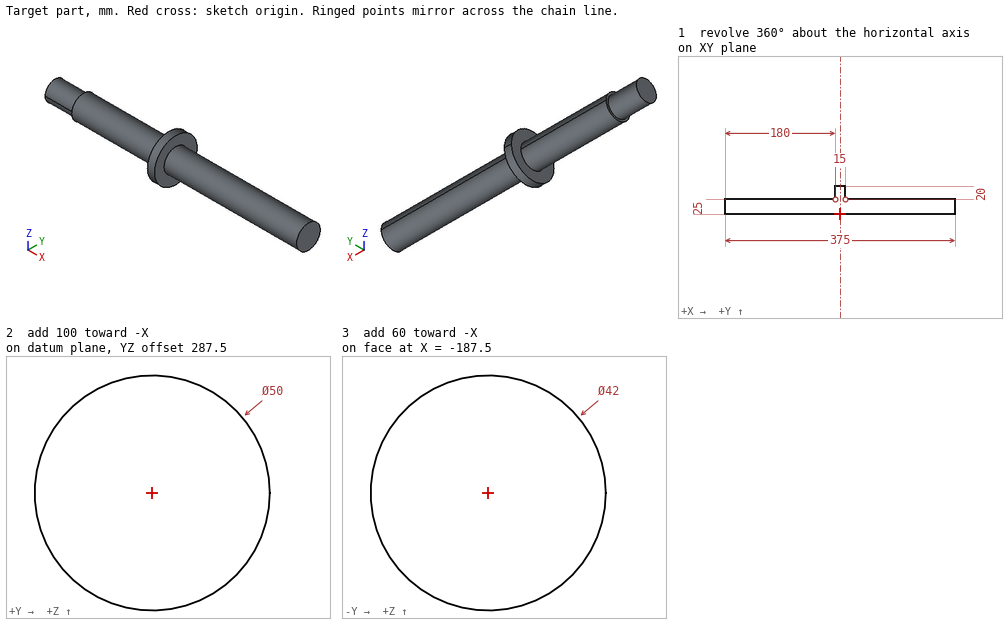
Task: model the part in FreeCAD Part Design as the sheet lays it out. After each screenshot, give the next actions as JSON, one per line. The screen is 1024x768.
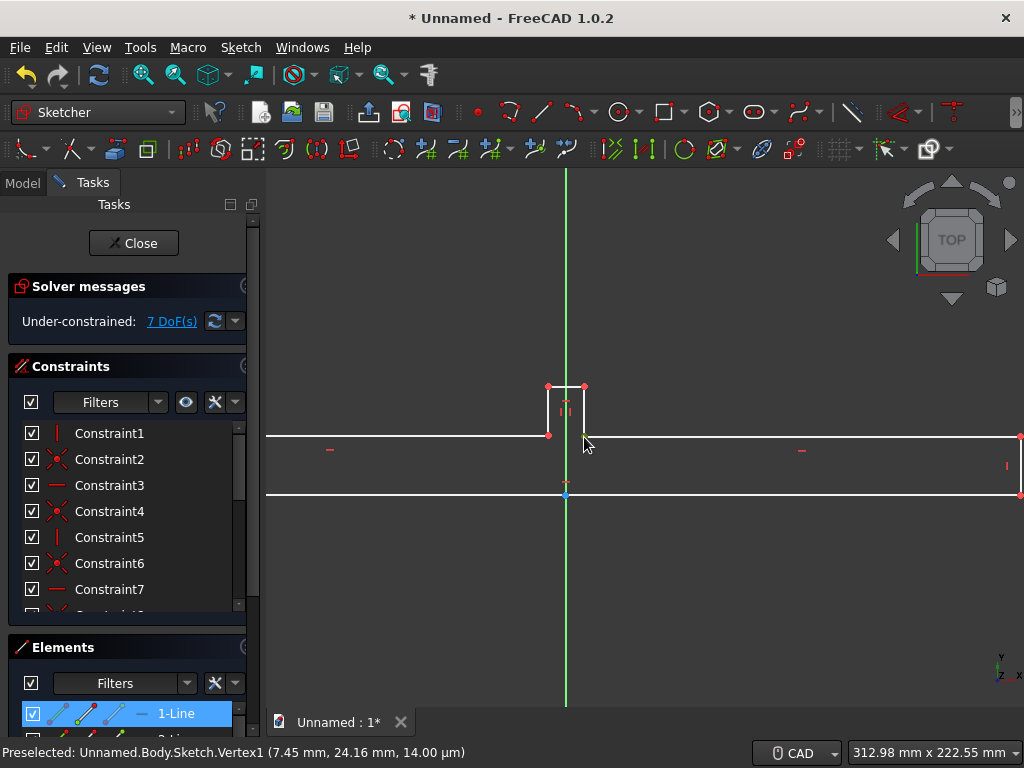
{"action": "left_click", "coordinate": [548, 436]}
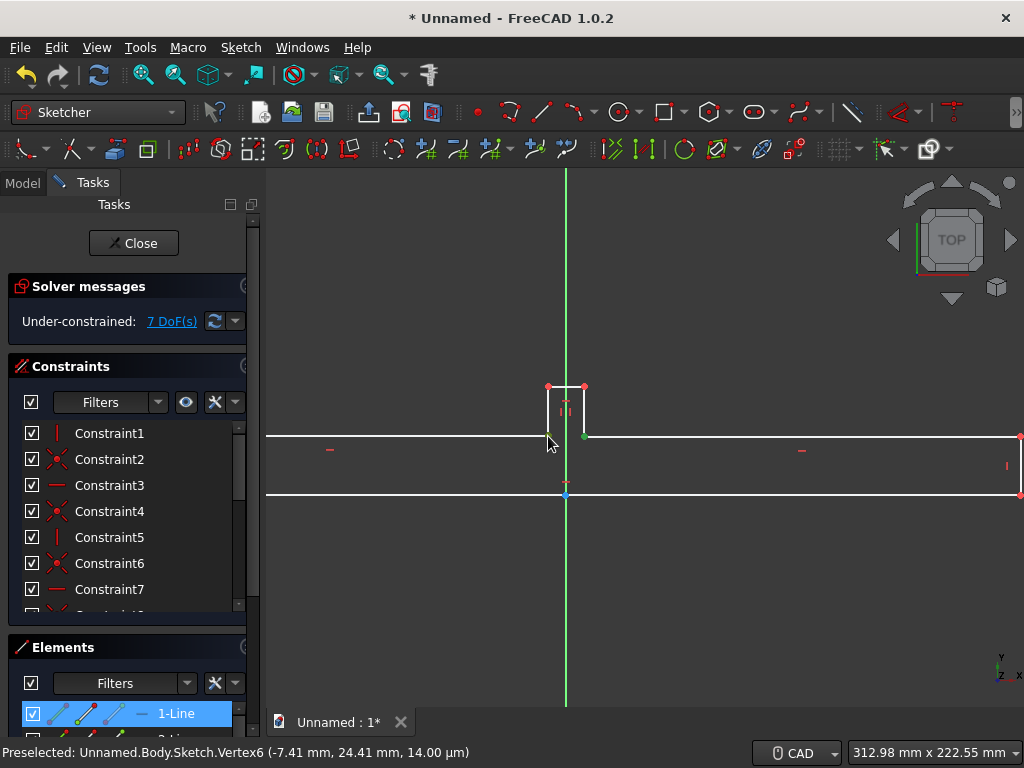
{"action": "left_click", "coordinate": [566, 644]}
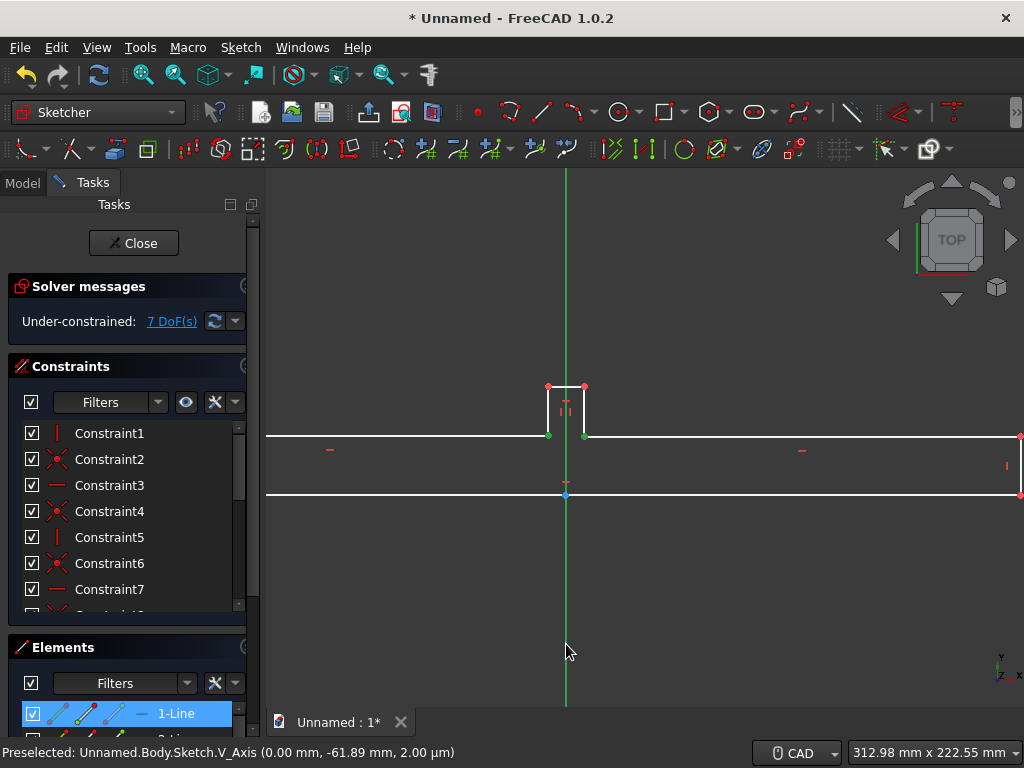
{"action": "key", "text": "s"}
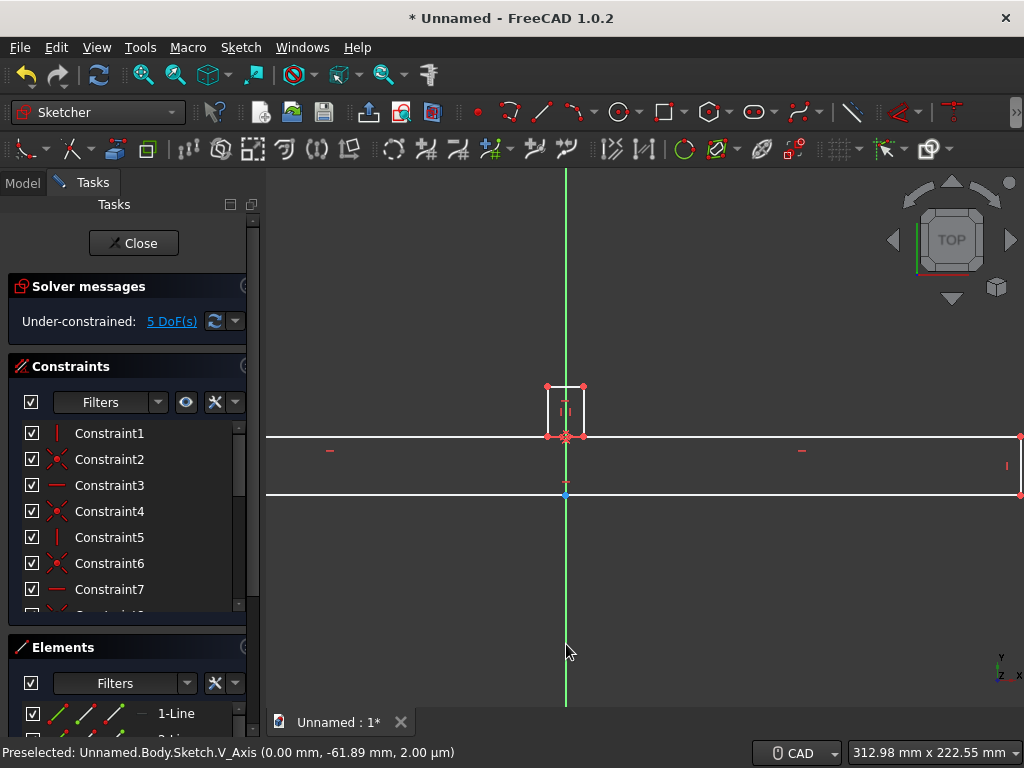
{"action": "left_click", "coordinate": [898, 112]}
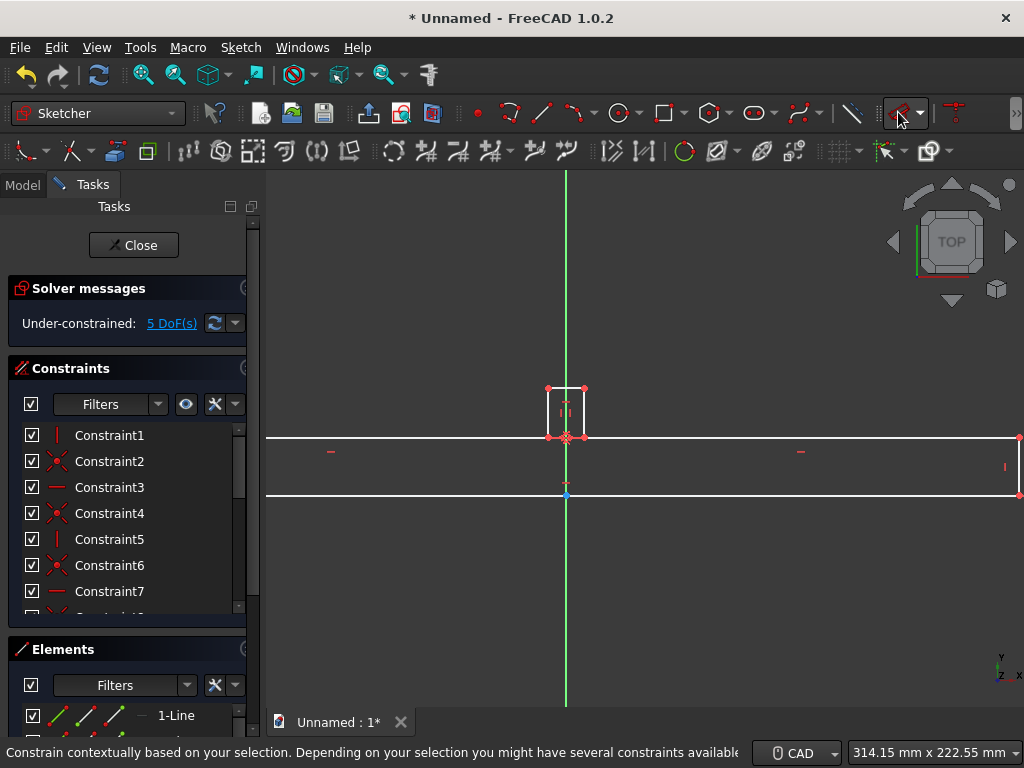
{"action": "left_click", "coordinate": [584, 423]}
{"action": "left_click", "coordinate": [618, 413]}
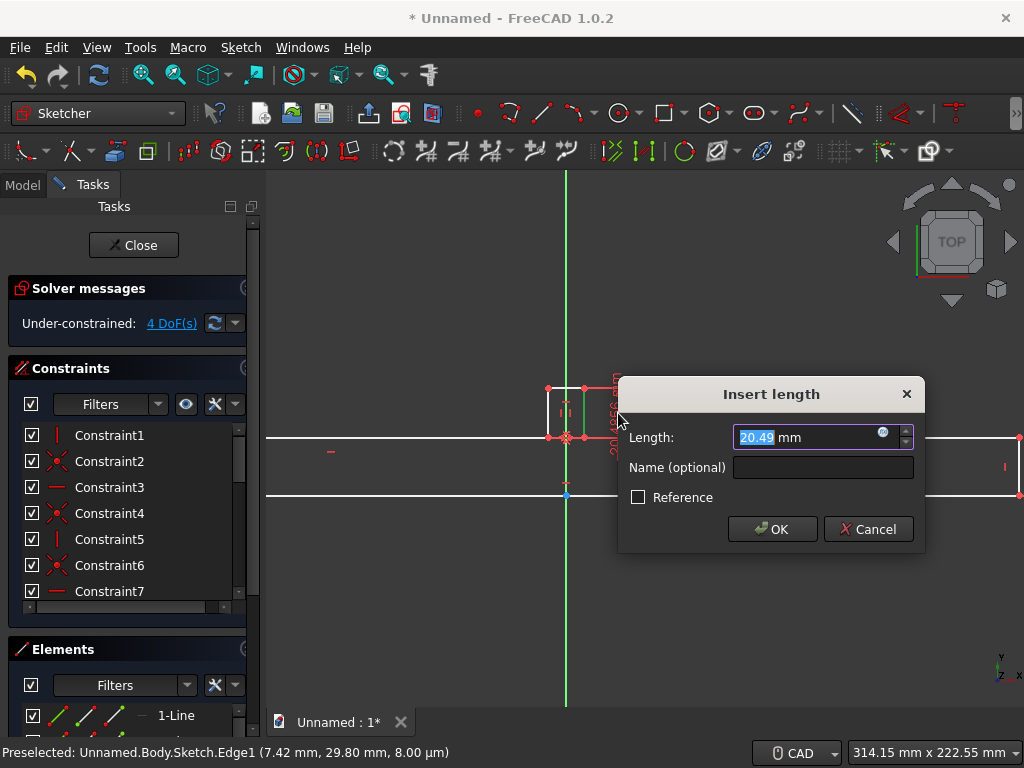
{"action": "type", "text": "20"}
{"action": "key", "text": "Return"}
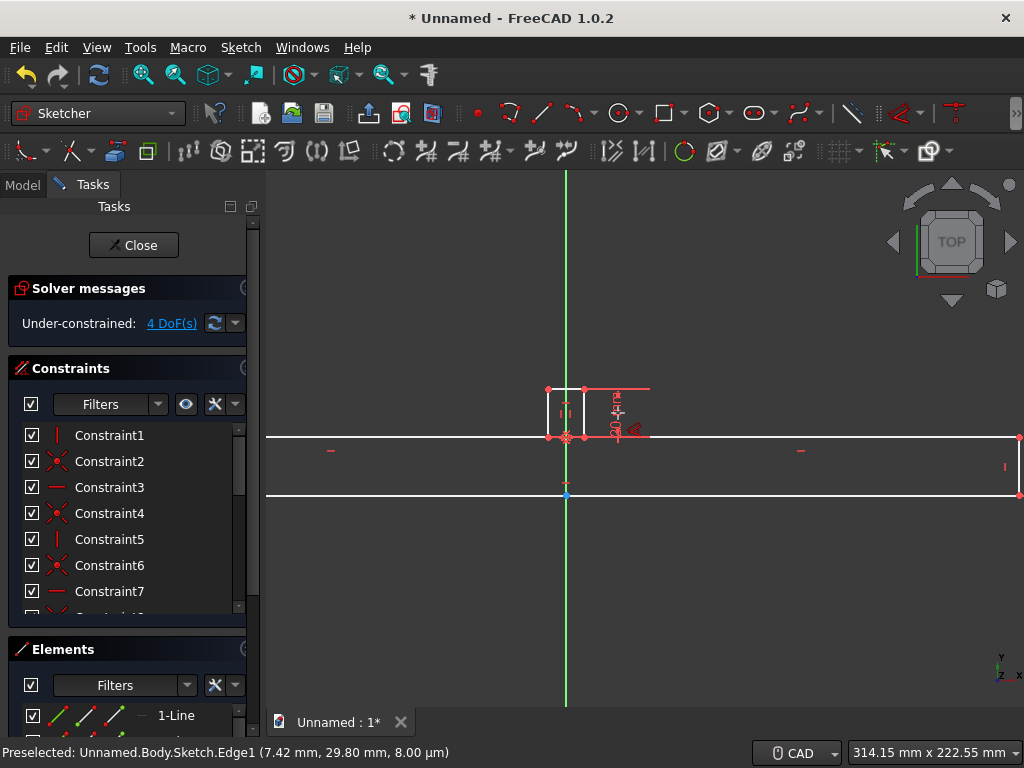
{"action": "left_click", "coordinate": [570, 389]}
{"action": "left_click", "coordinate": [558, 355]}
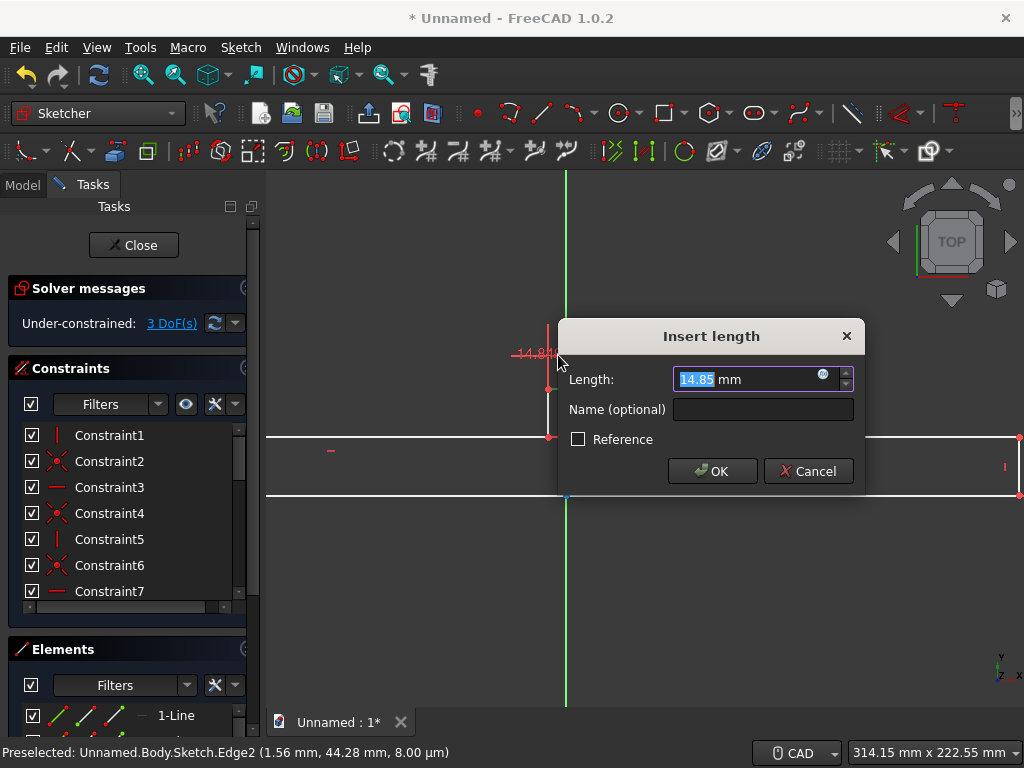
{"action": "type", "text": "15"}
{"action": "key", "text": "Return"}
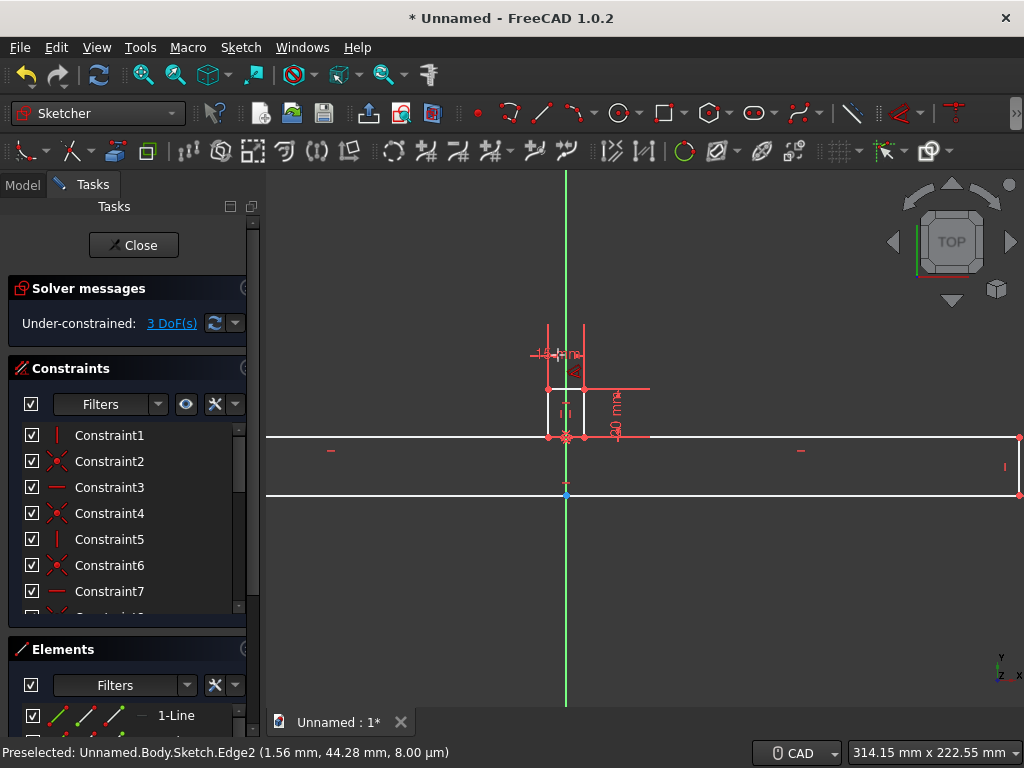
{"action": "scroll", "coordinate": [585, 436], "scroll_direction": "down", "scroll_amount": 4}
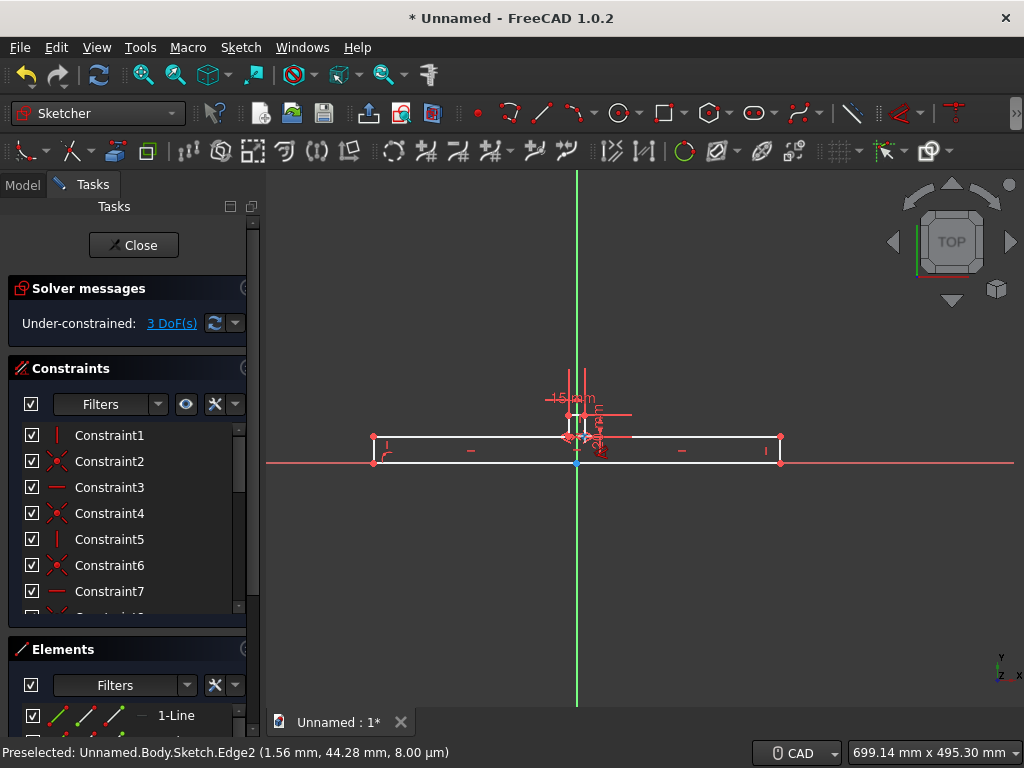
{"action": "scroll", "coordinate": [374, 445], "scroll_direction": "up", "scroll_amount": 3}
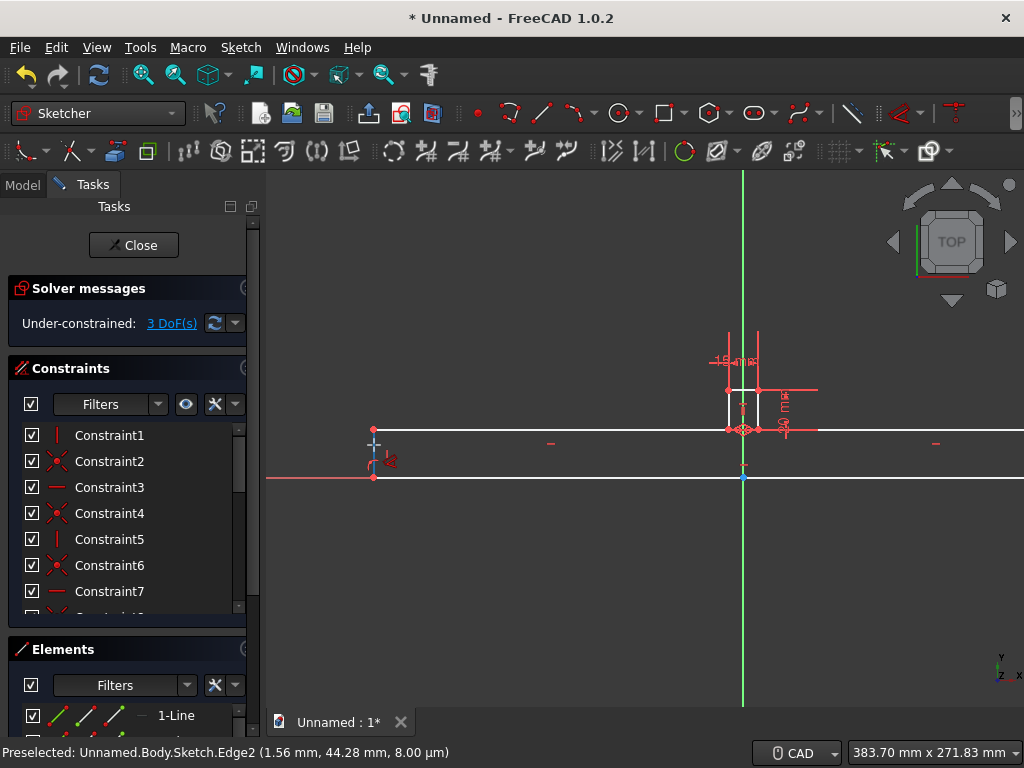
{"action": "left_click", "coordinate": [374, 444]}
{"action": "left_click", "coordinate": [340, 454]}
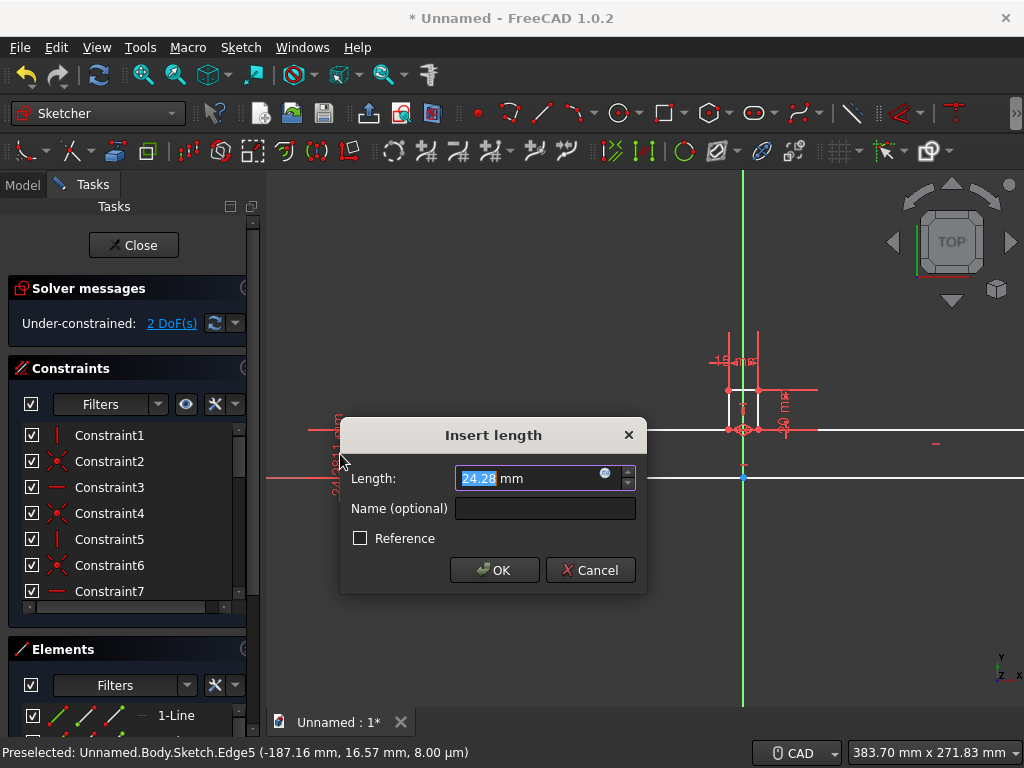
{"action": "type", "text": "25"}
{"action": "key", "text": "Return"}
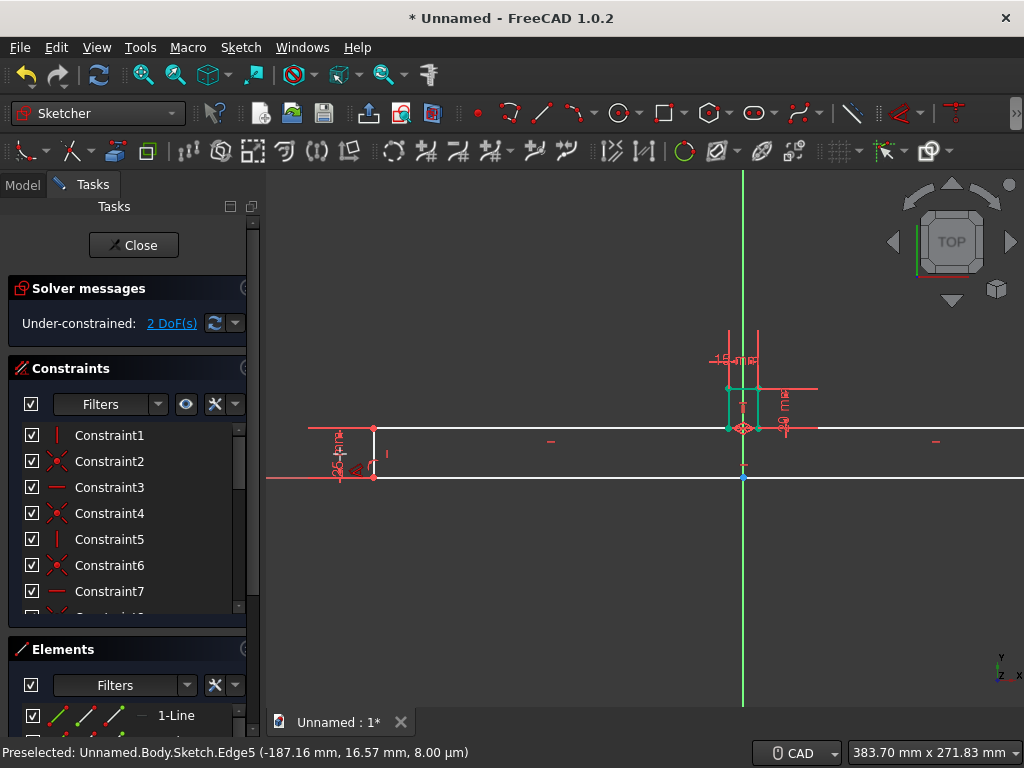
{"action": "left_click", "coordinate": [622, 428]}
{"action": "left_click", "coordinate": [551, 394]}